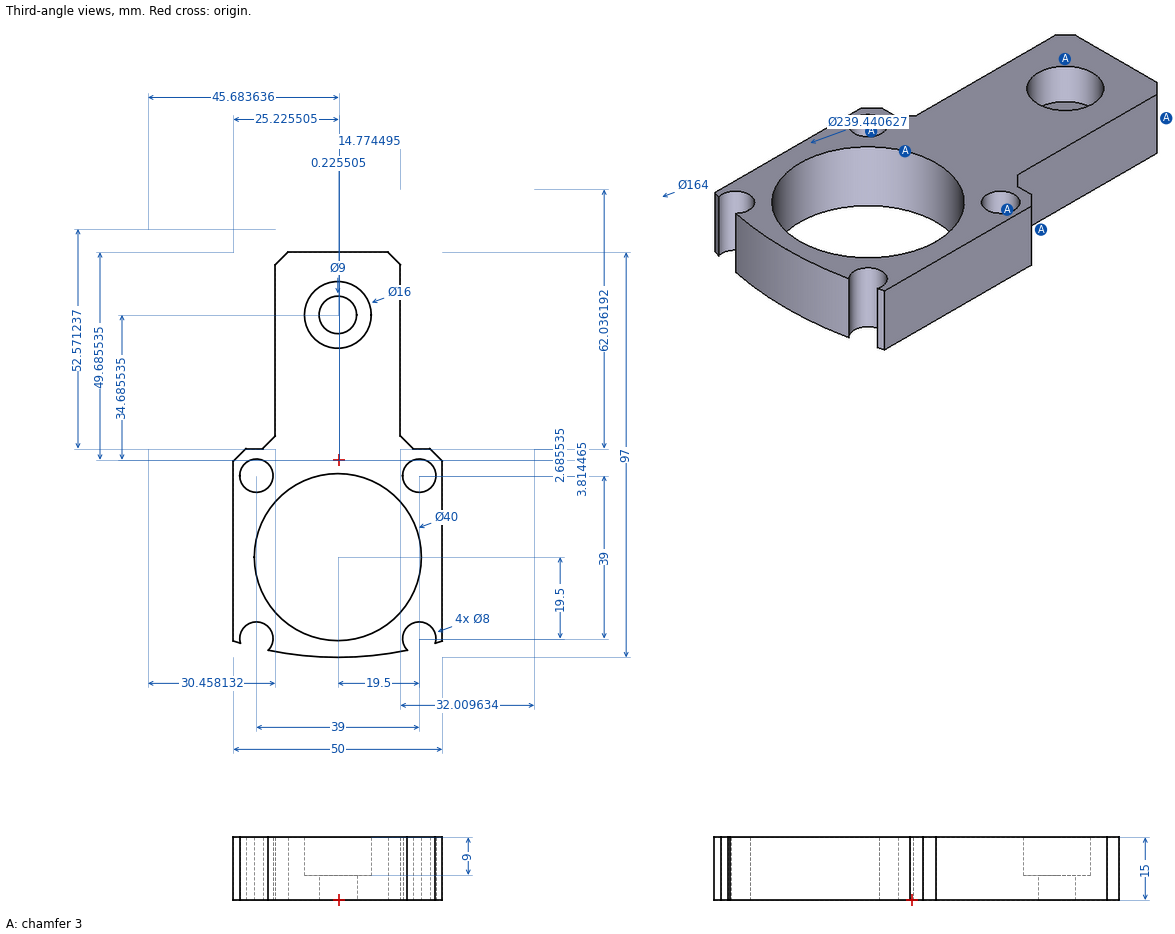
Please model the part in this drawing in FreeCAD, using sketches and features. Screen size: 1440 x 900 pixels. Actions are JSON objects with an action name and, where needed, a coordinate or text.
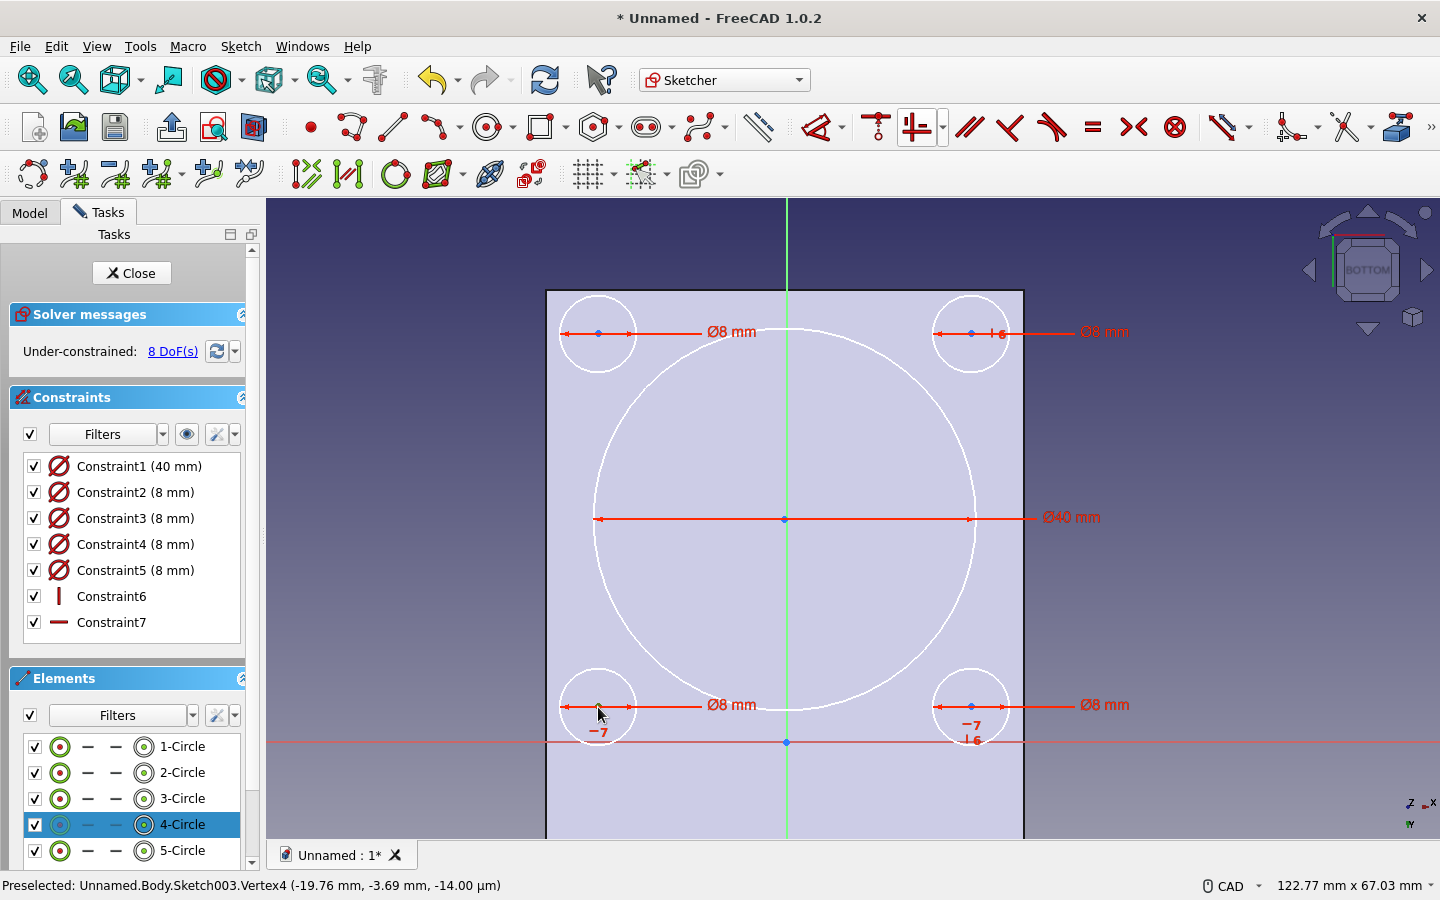
{"action": "left_click", "coordinate": [598, 334]}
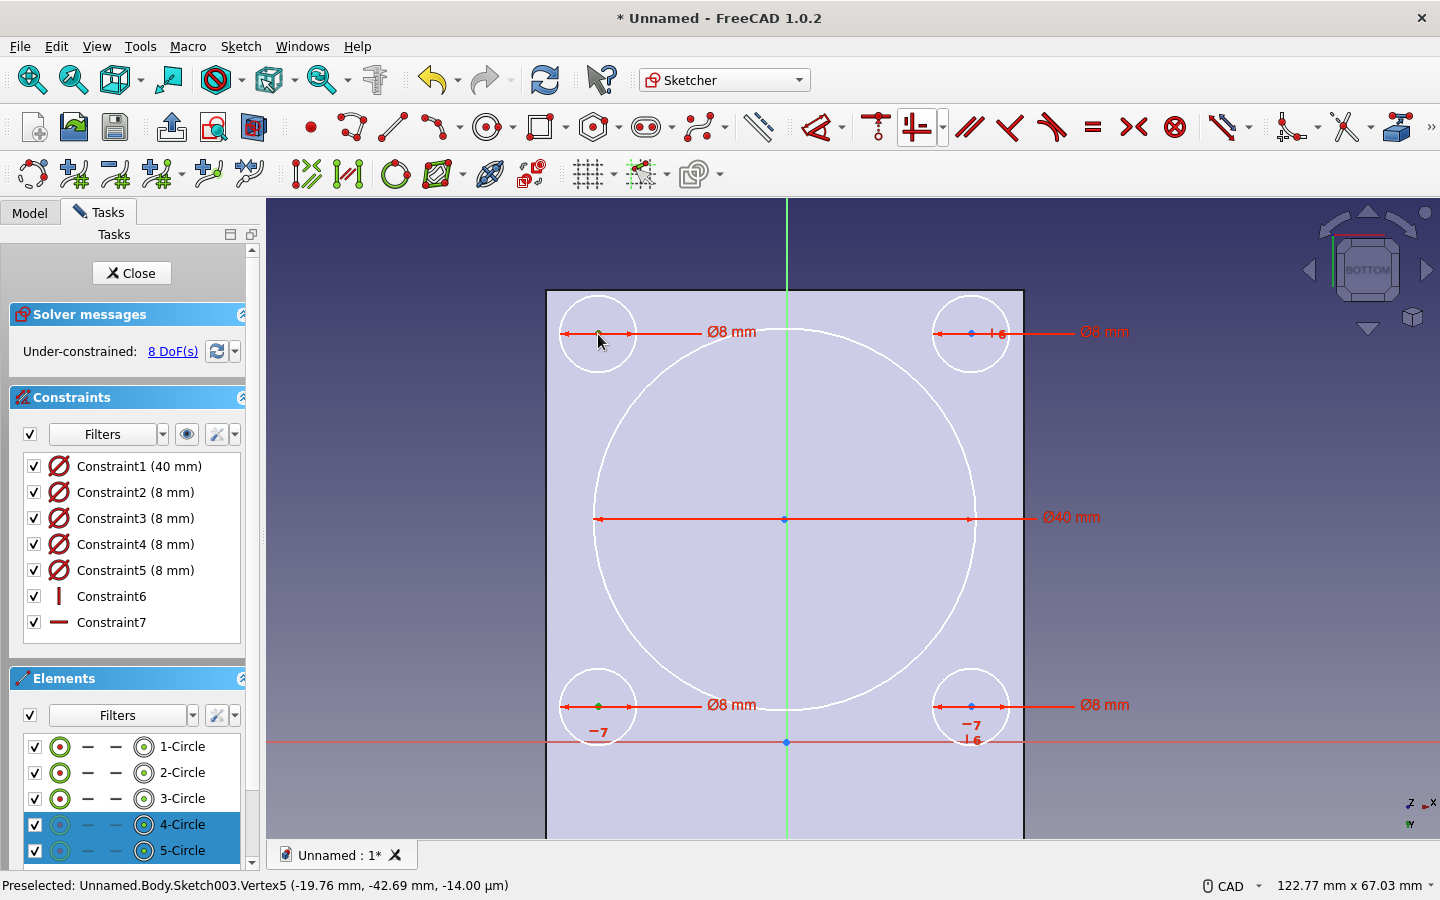
{"action": "key", "text": "v"}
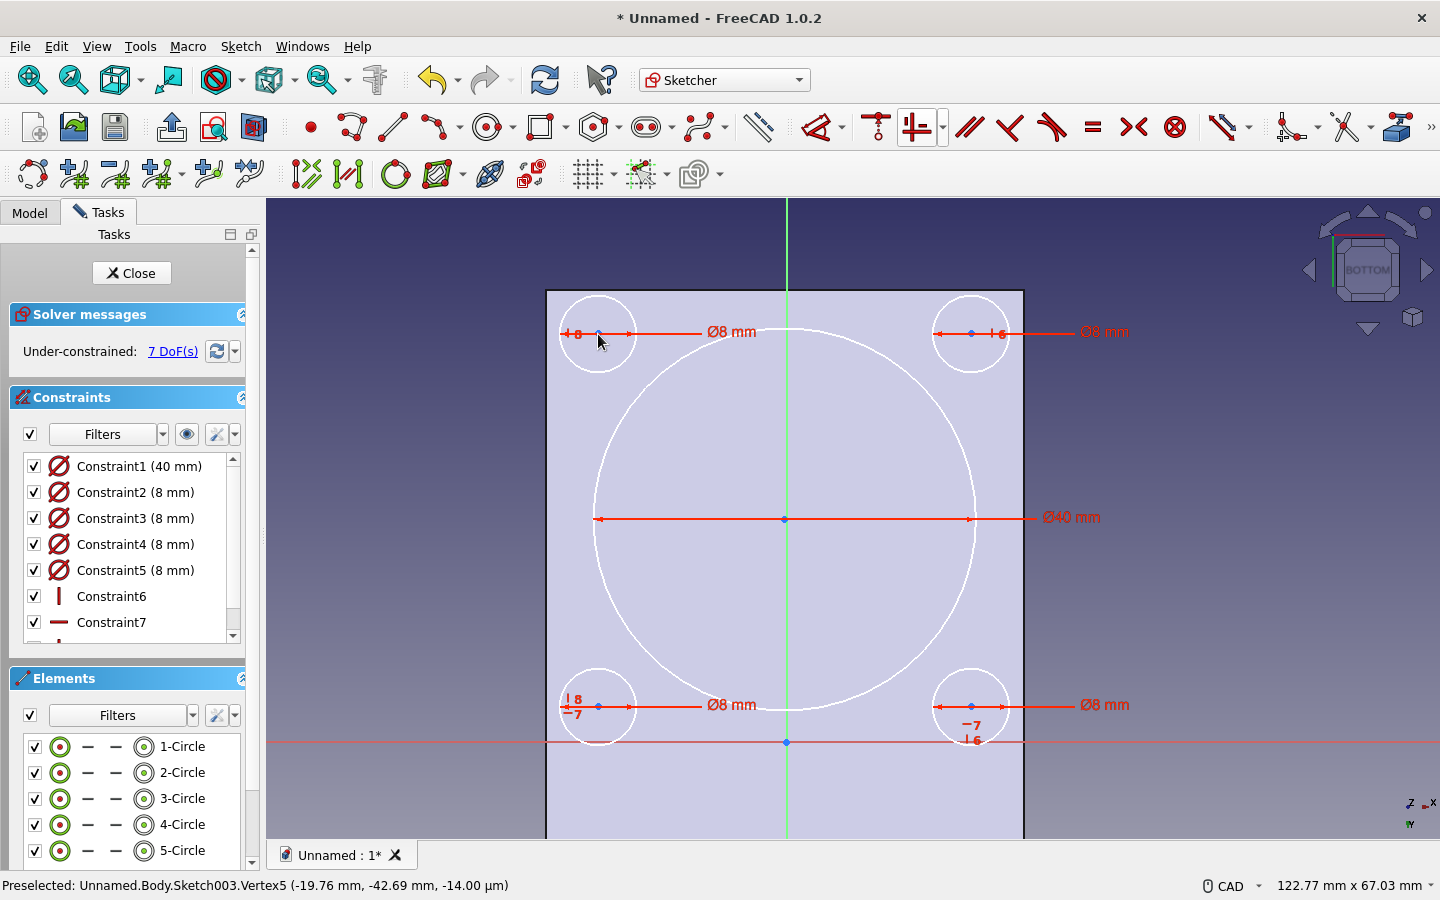
{"action": "left_click", "coordinate": [971, 334]}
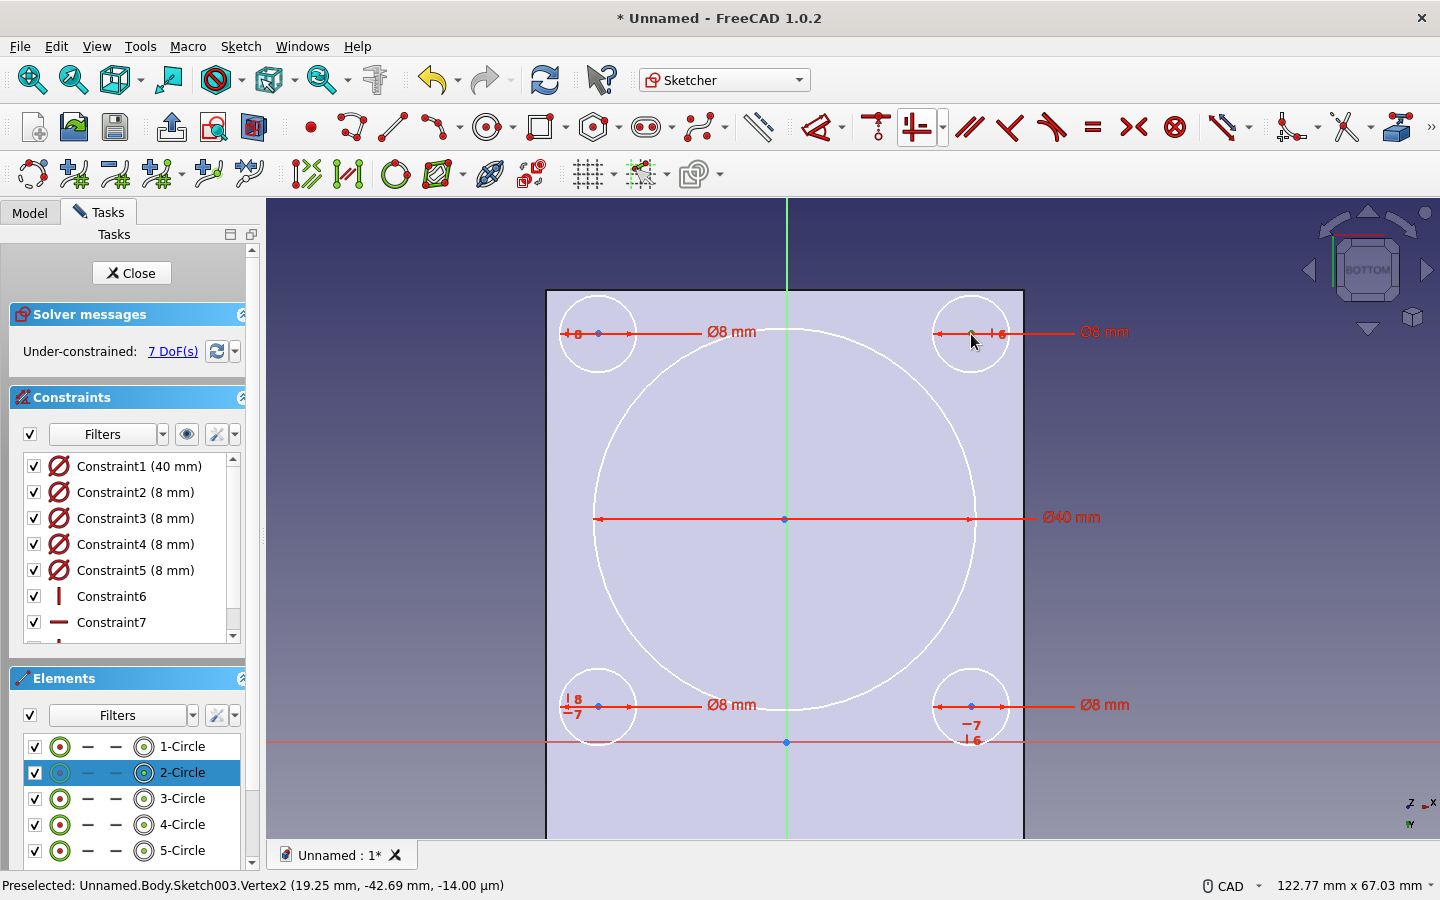
{"action": "left_click", "coordinate": [598, 334]}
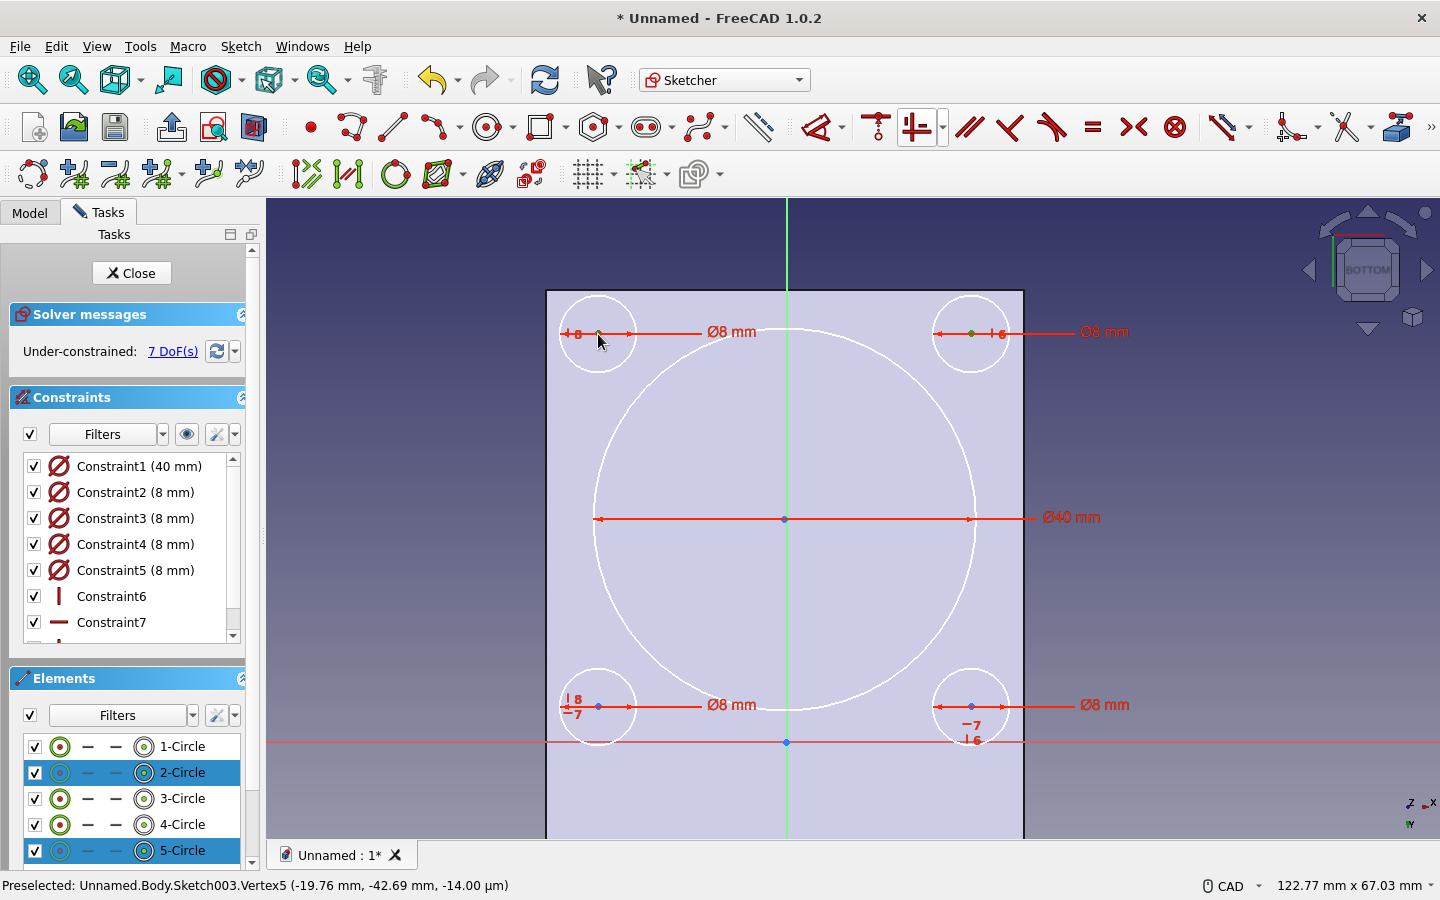
{"action": "left_click", "coordinate": [942, 128]}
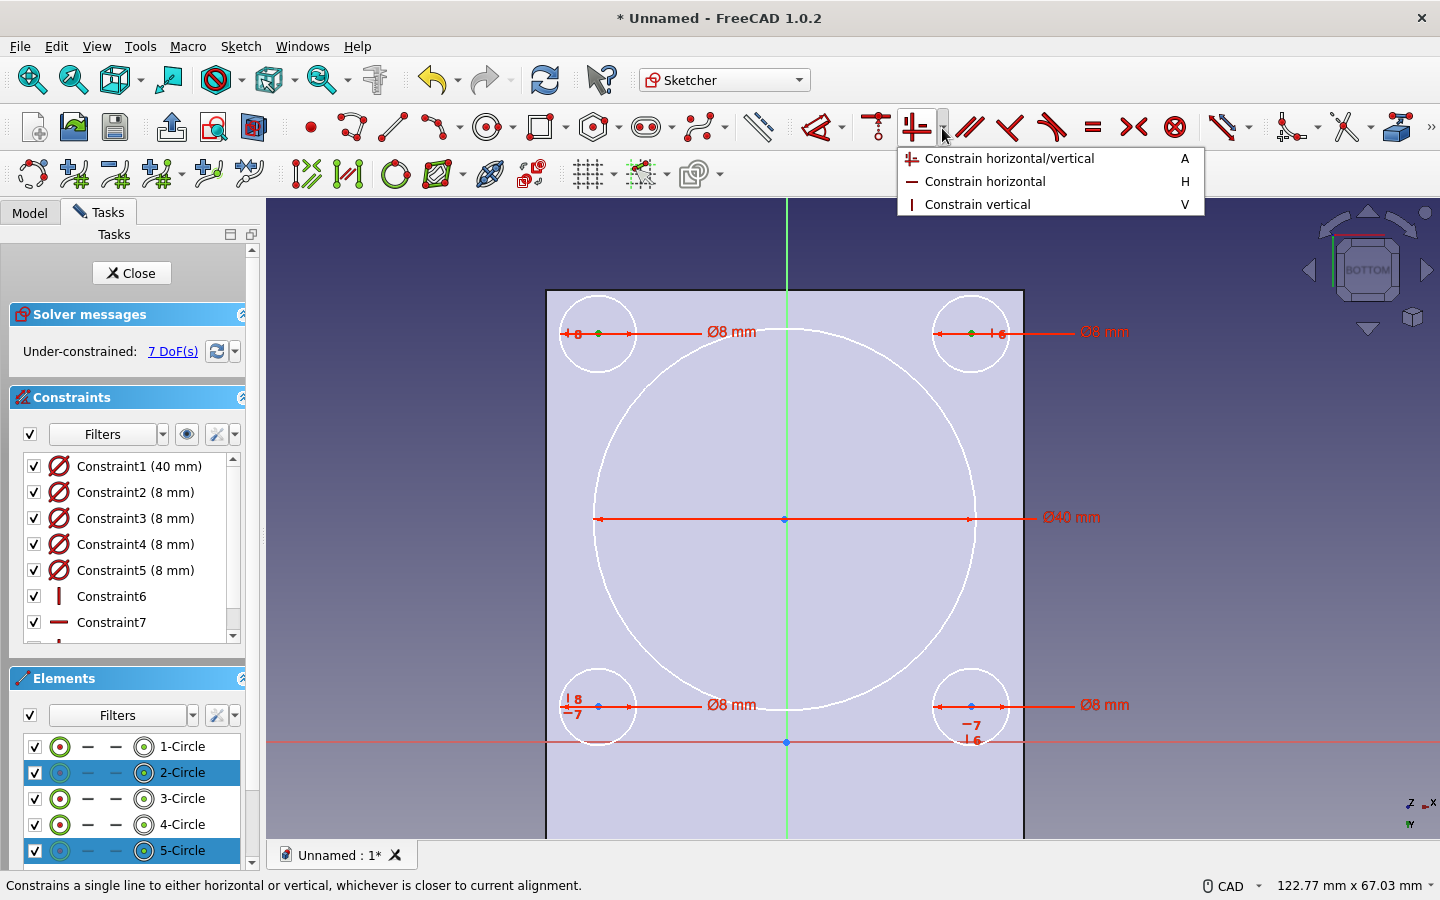
{"action": "left_click", "coordinate": [1051, 182]}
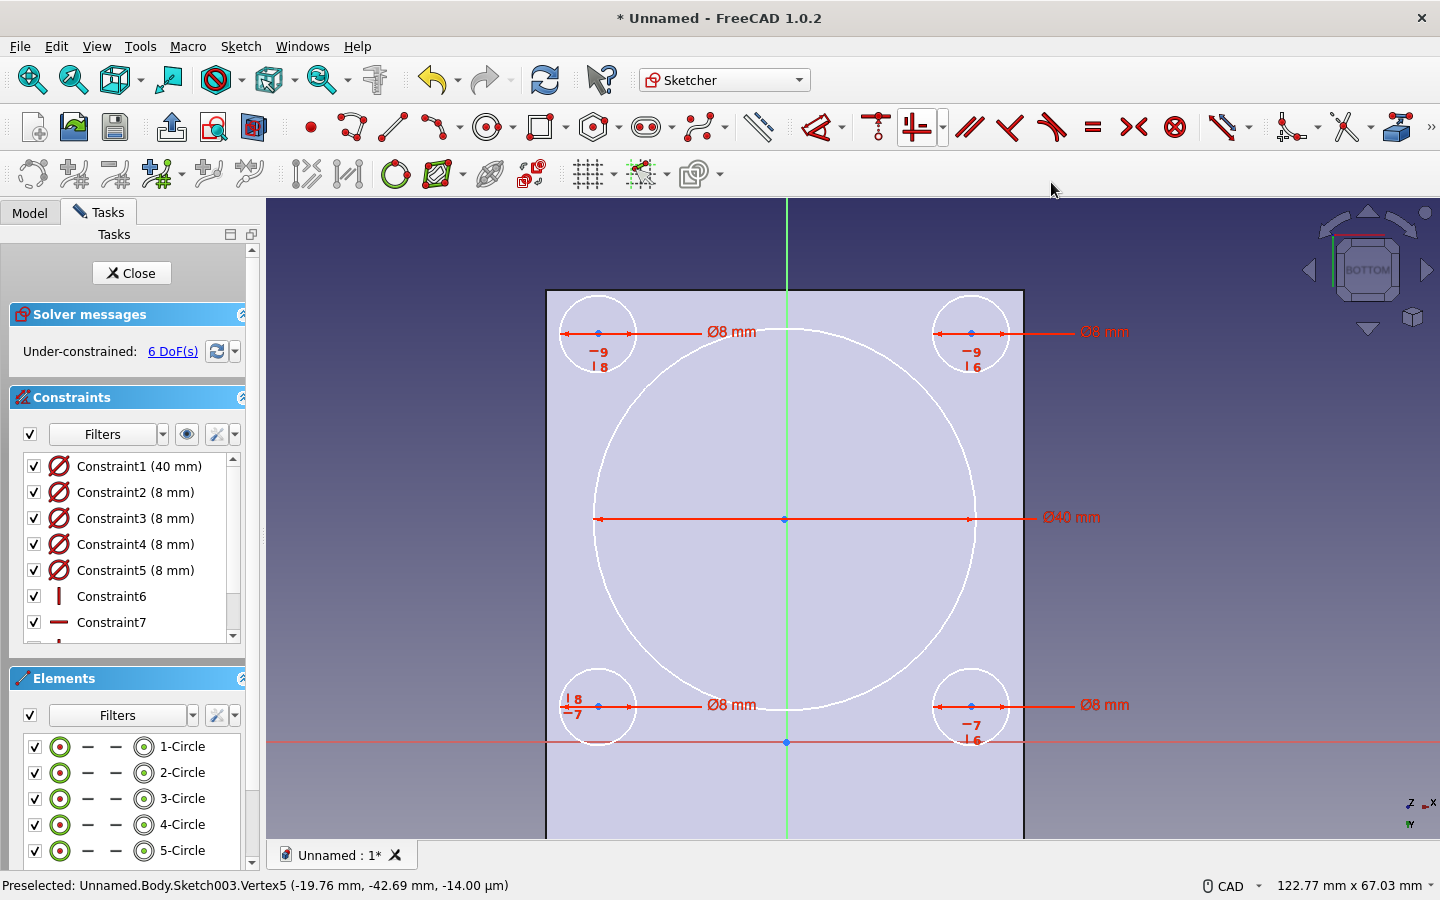
{"action": "key", "text": "d"}